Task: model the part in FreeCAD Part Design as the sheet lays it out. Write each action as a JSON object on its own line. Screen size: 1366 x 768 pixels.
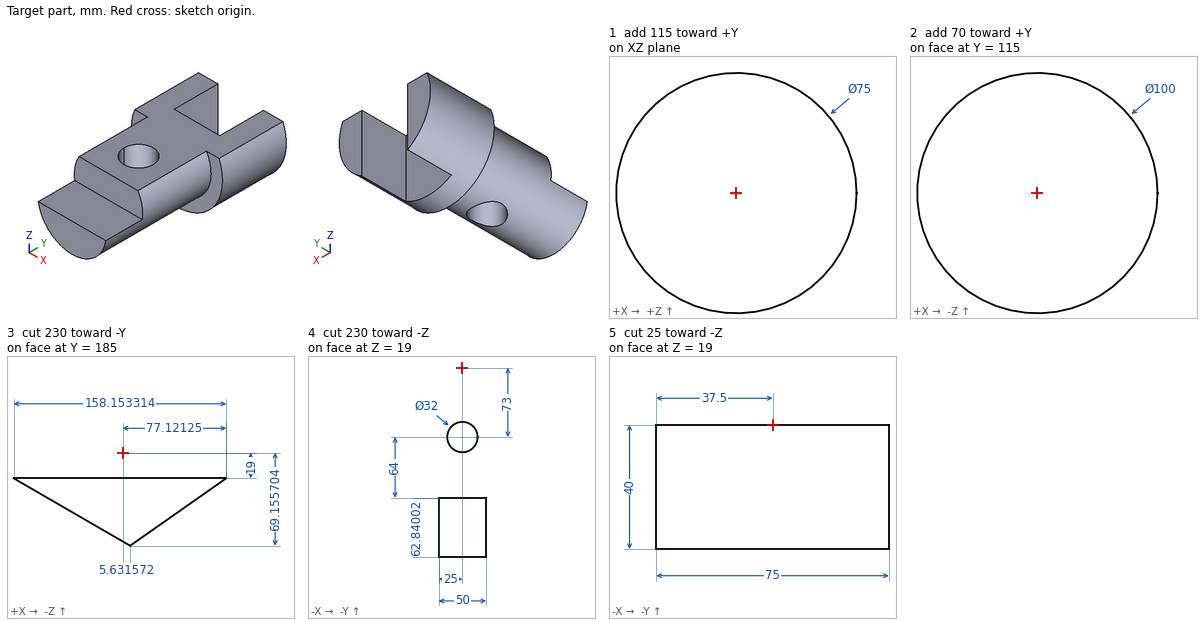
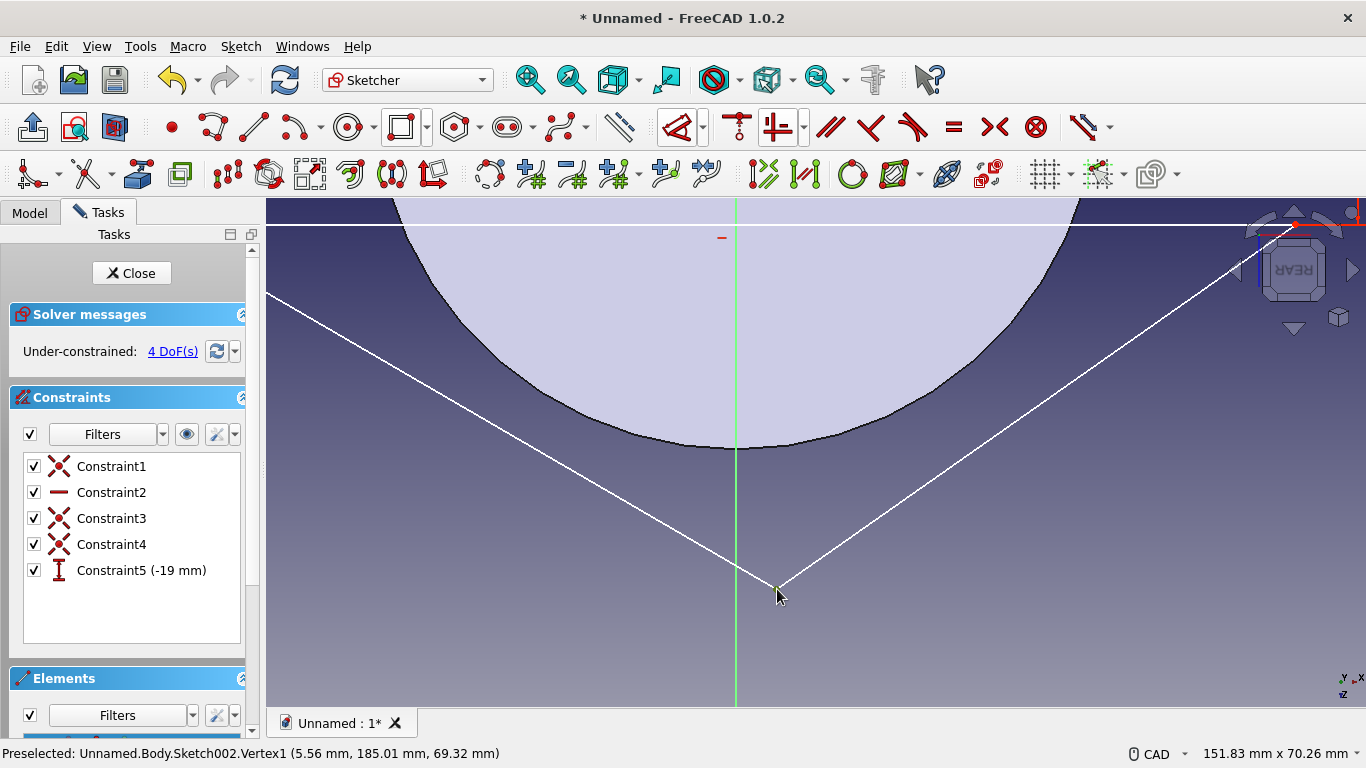
{"action": "left_click", "coordinate": [702, 128]}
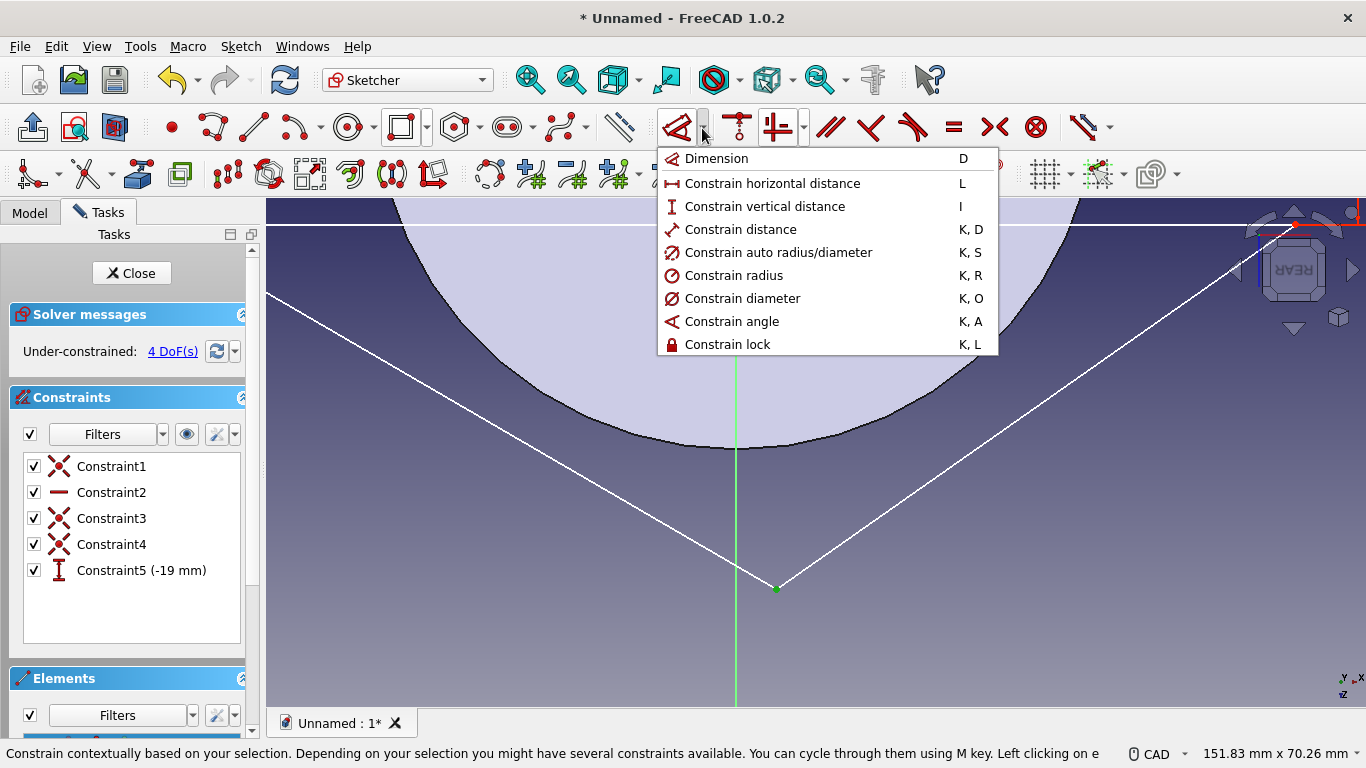
{"action": "left_click", "coordinate": [828, 184]}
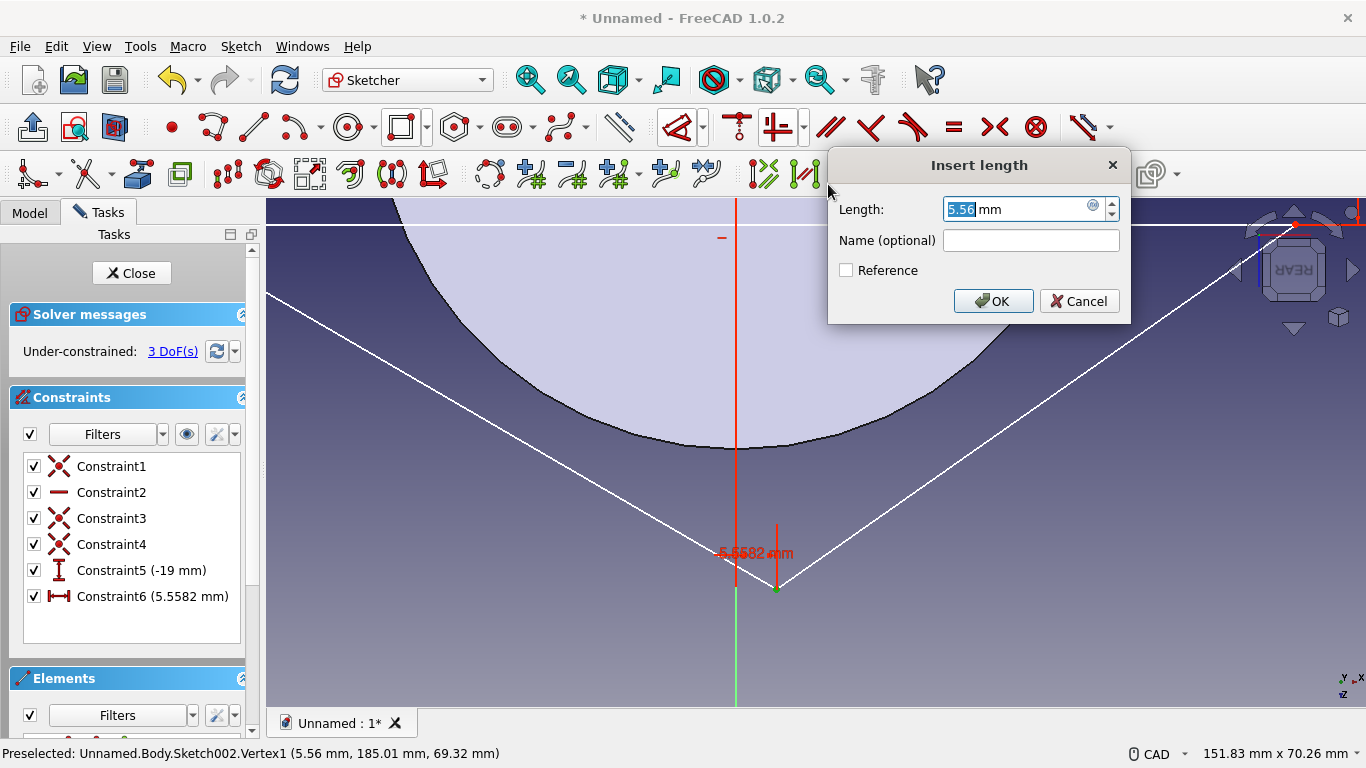
{"action": "type", "text": "5.631572"}
{"action": "key", "text": "Return"}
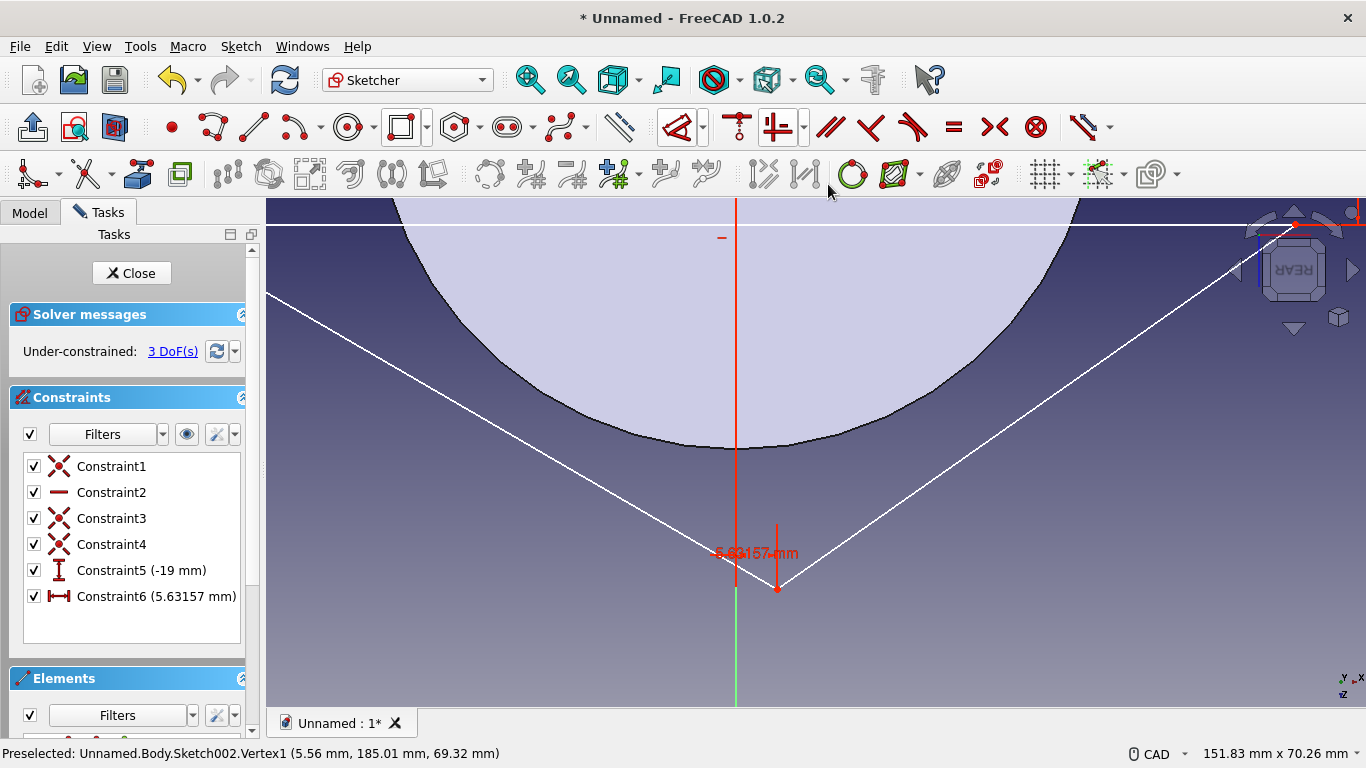
{"action": "scroll", "coordinate": [778, 592], "scroll_direction": "down", "scroll_amount": 3}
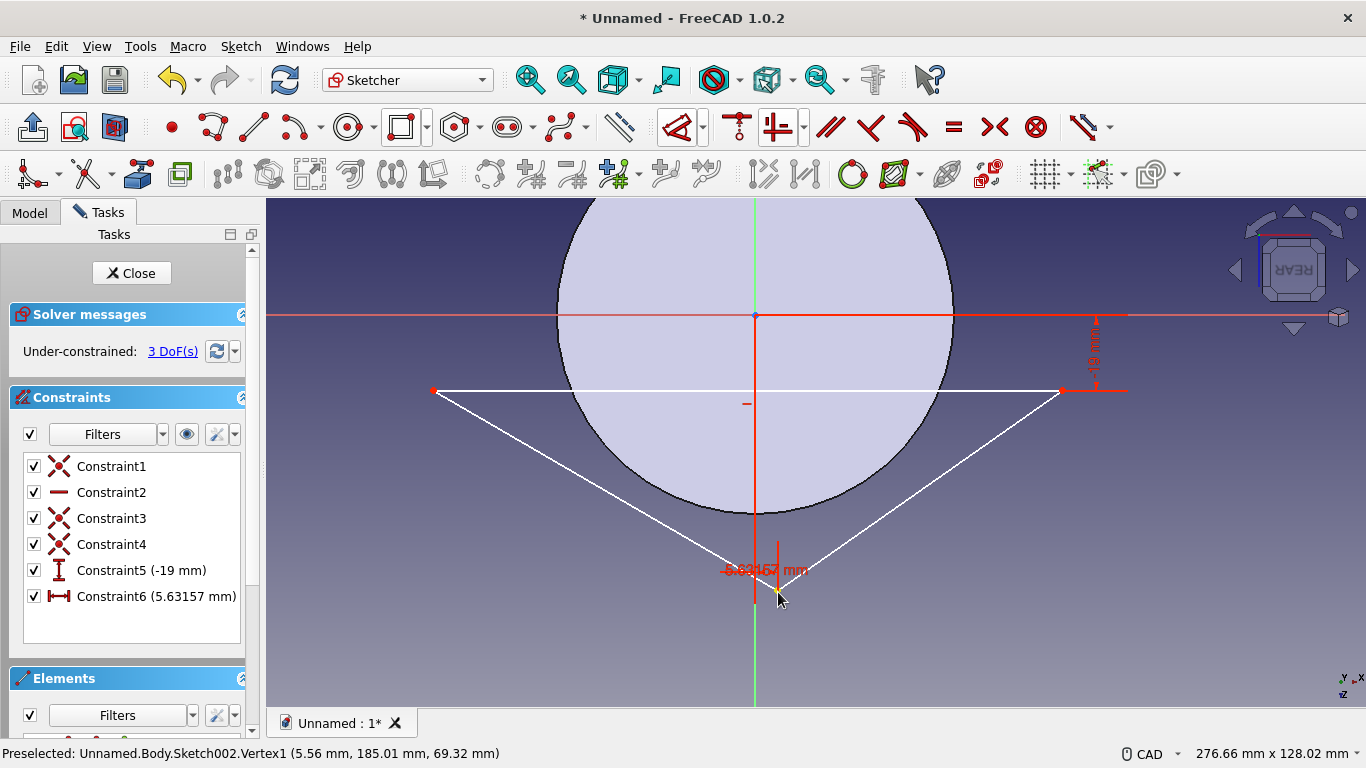
{"action": "left_click", "coordinate": [1062, 391]}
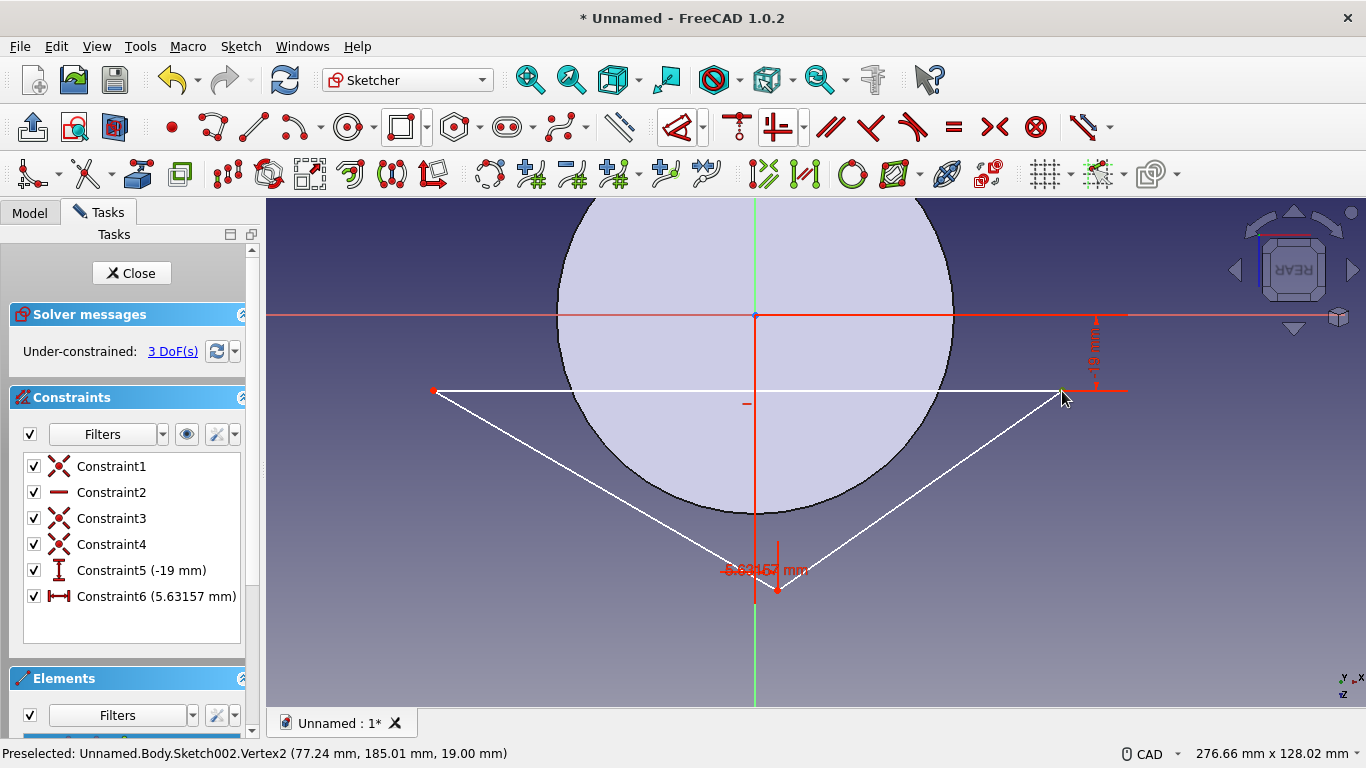
{"action": "key", "text": "l"}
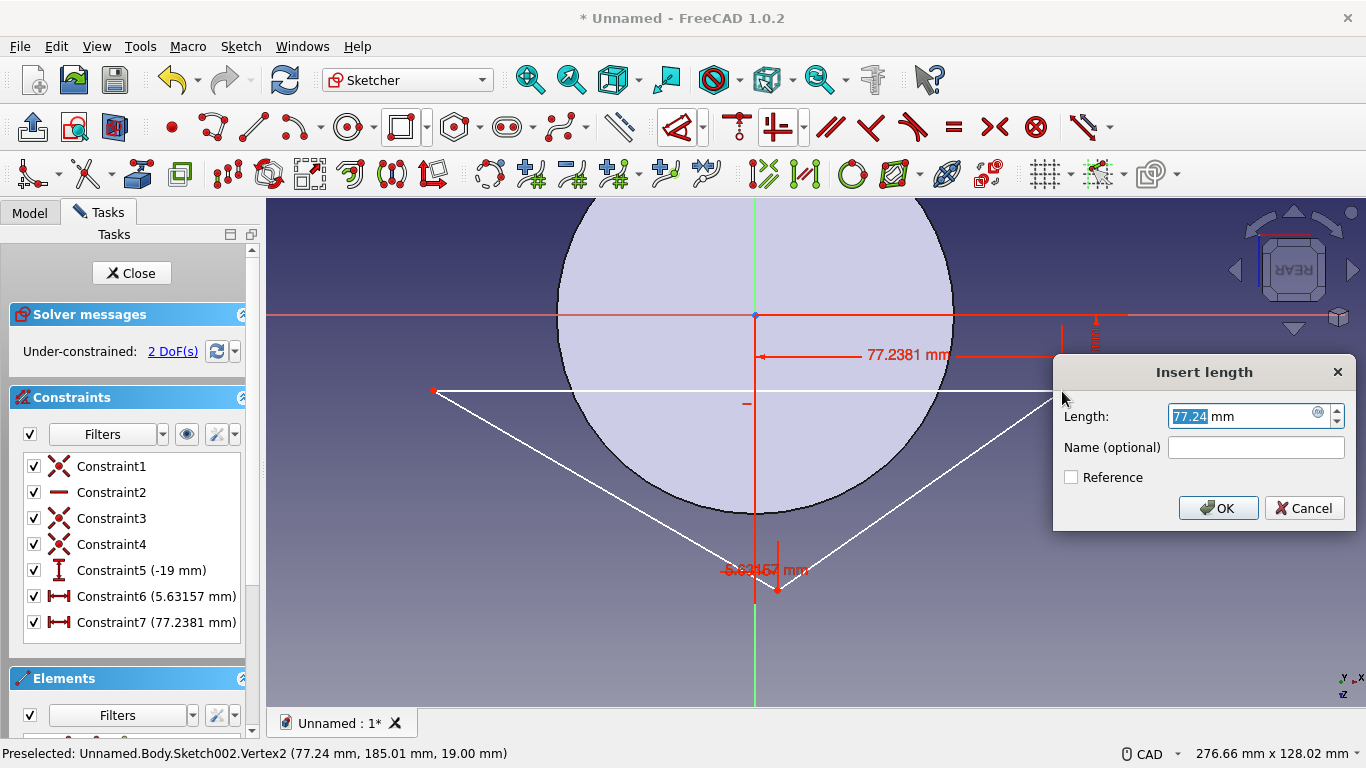
{"action": "type", "text": "77.12125"}
{"action": "key", "text": "Return"}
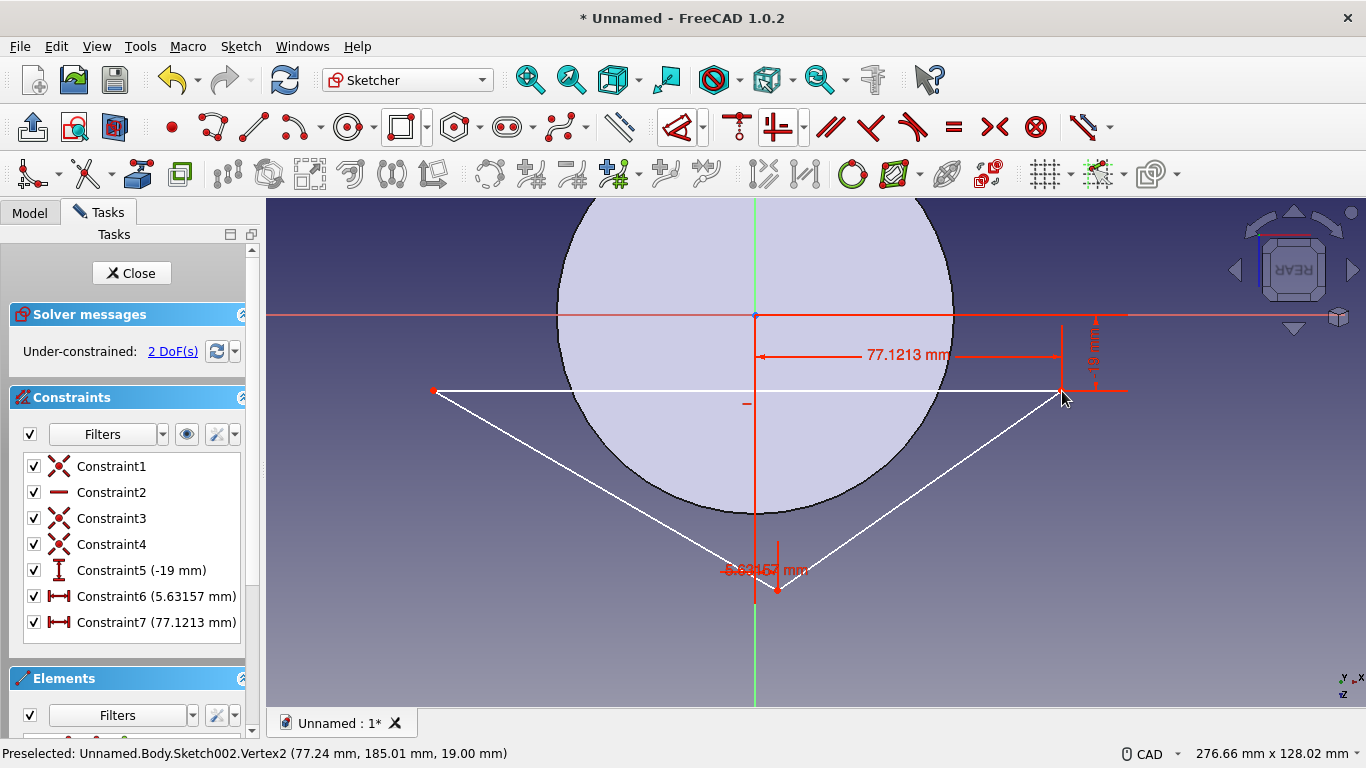
{"action": "left_click", "coordinate": [873, 391]}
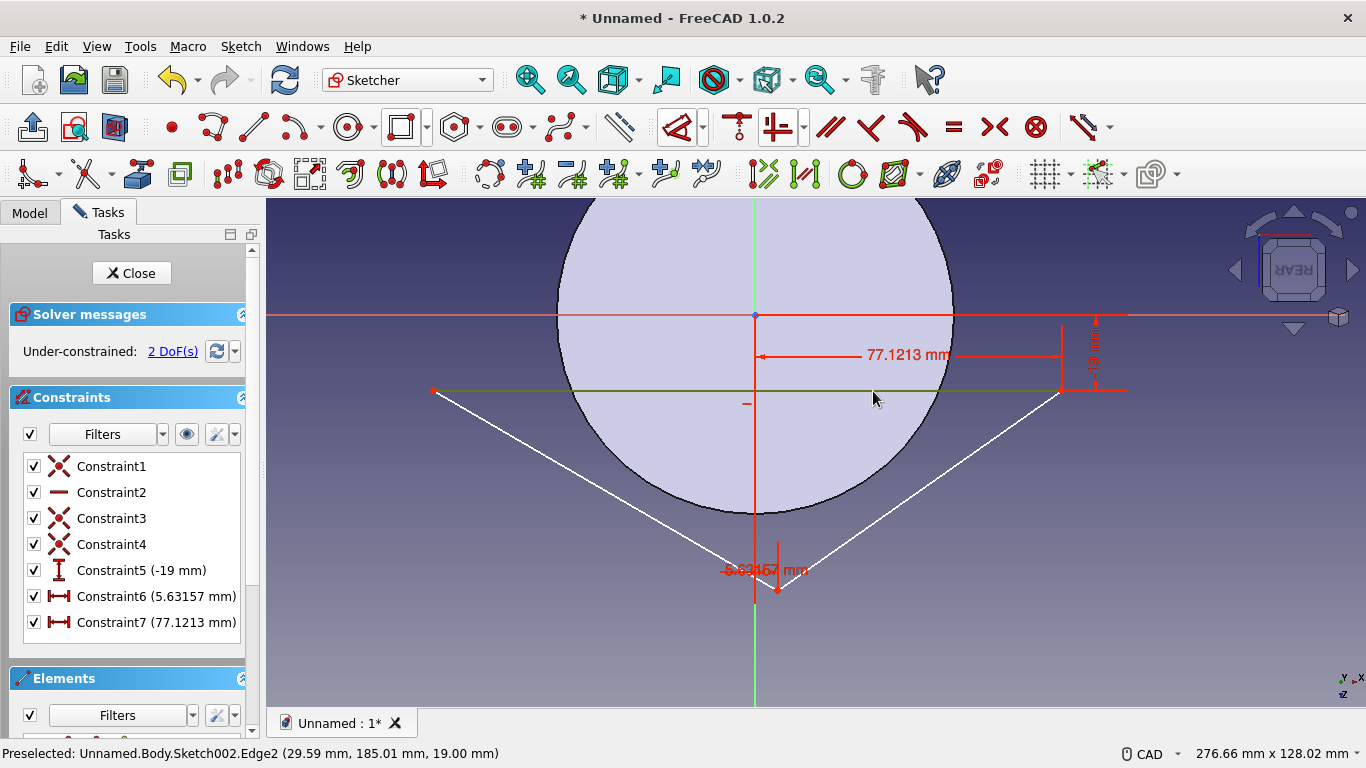
{"action": "left_click", "coordinate": [702, 128]}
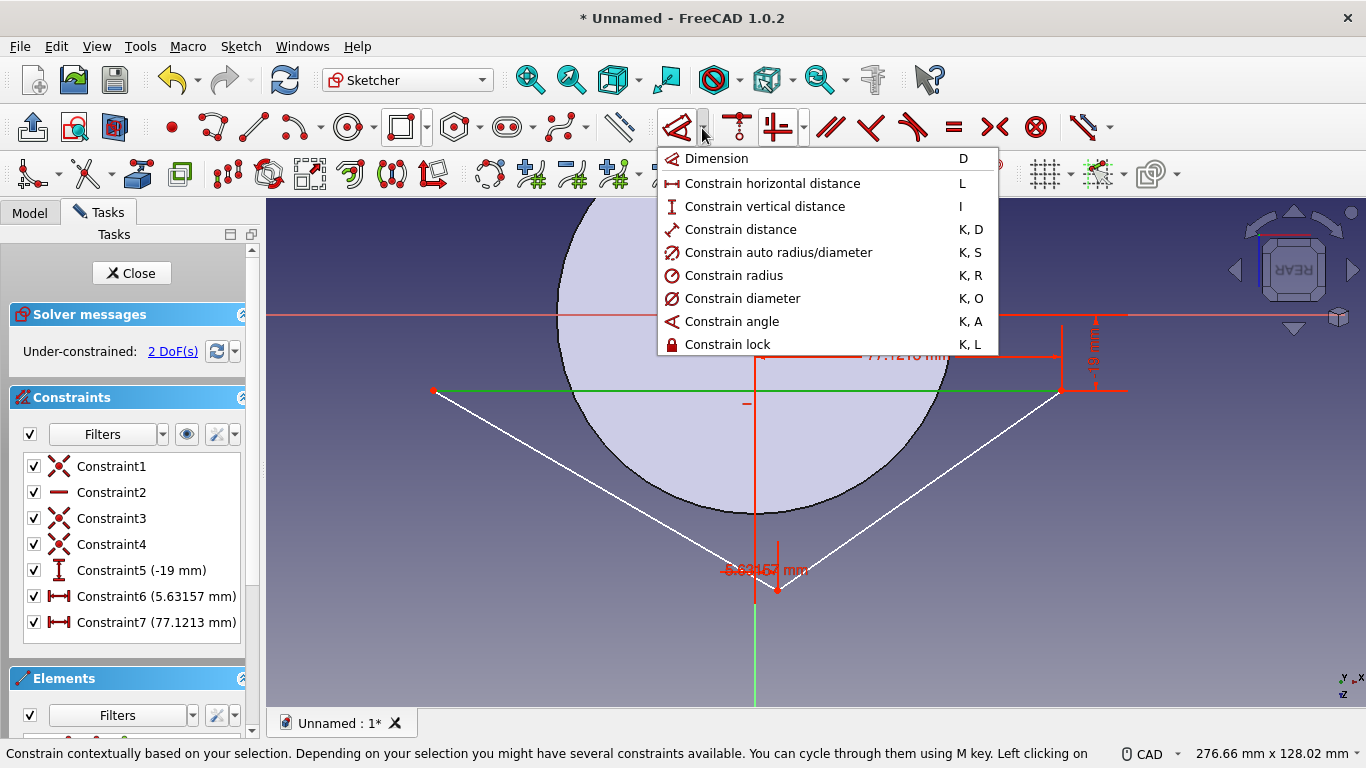
{"action": "left_click", "coordinate": [828, 184]}